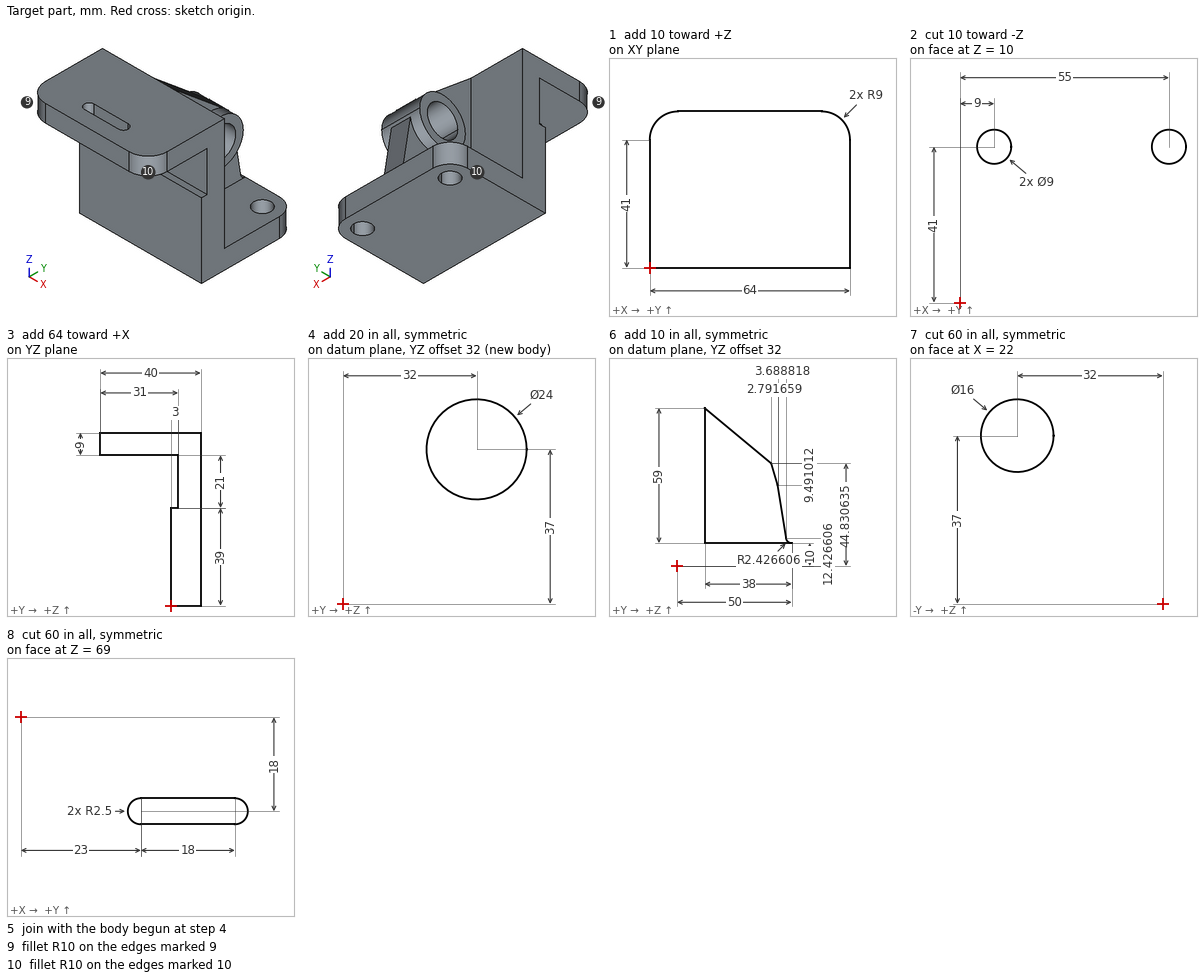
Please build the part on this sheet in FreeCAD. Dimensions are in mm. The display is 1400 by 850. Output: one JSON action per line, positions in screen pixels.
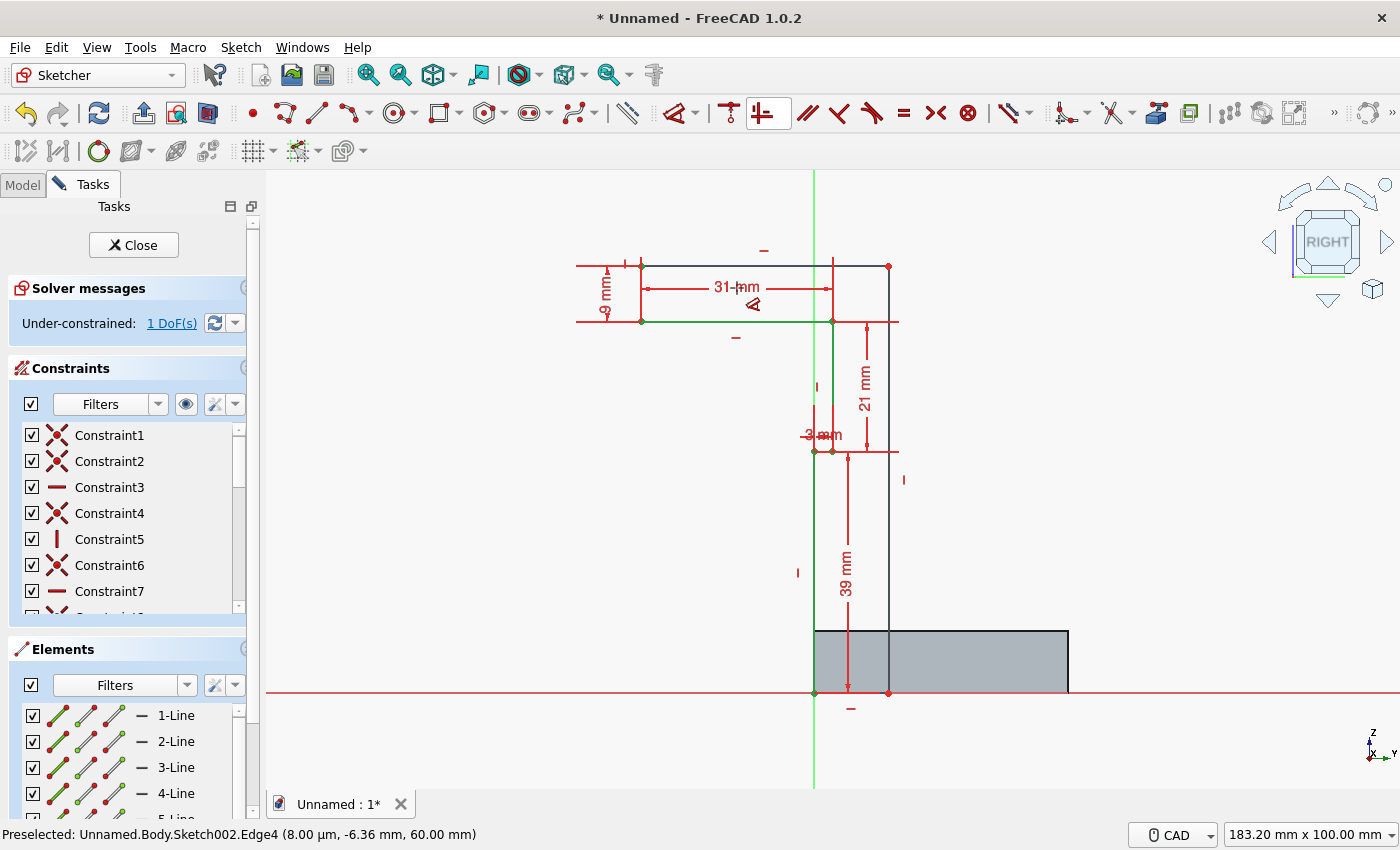
{"action": "left_click", "coordinate": [715, 266]}
{"action": "left_click", "coordinate": [765, 232]}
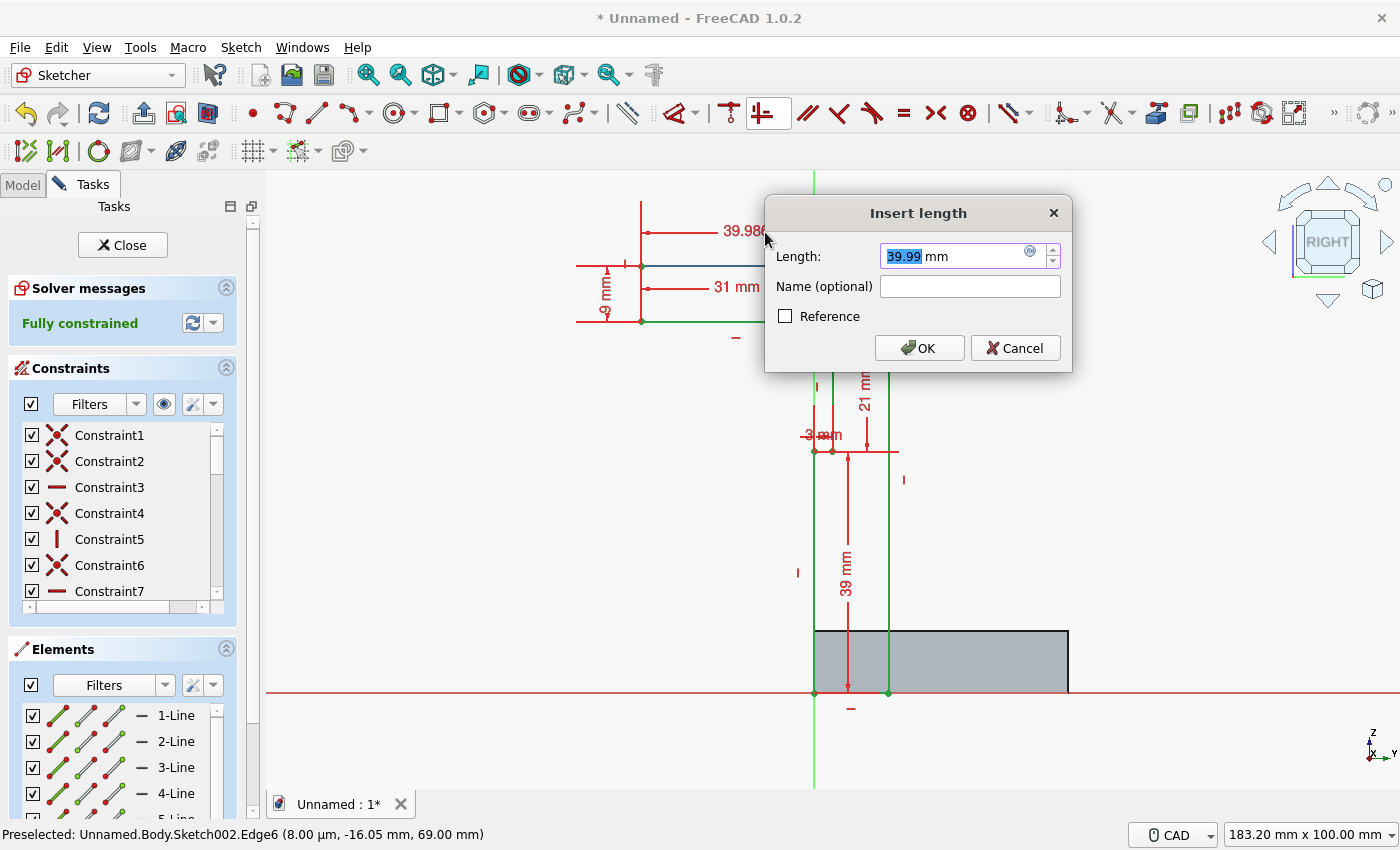
{"action": "type", "text": "40"}
{"action": "key", "text": "Return"}
{"action": "key", "text": "Escape"}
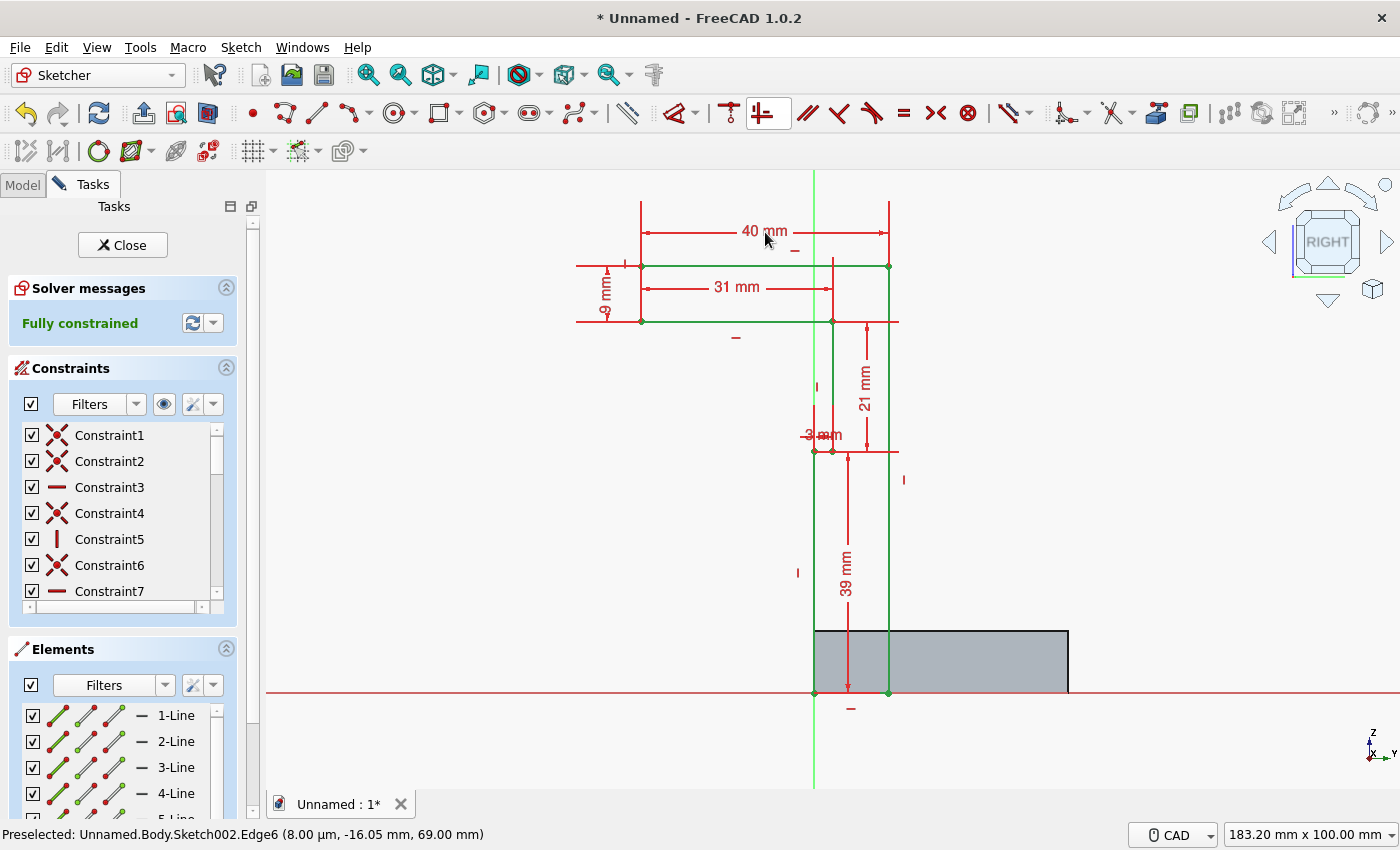
{"action": "left_click", "coordinate": [123, 245]}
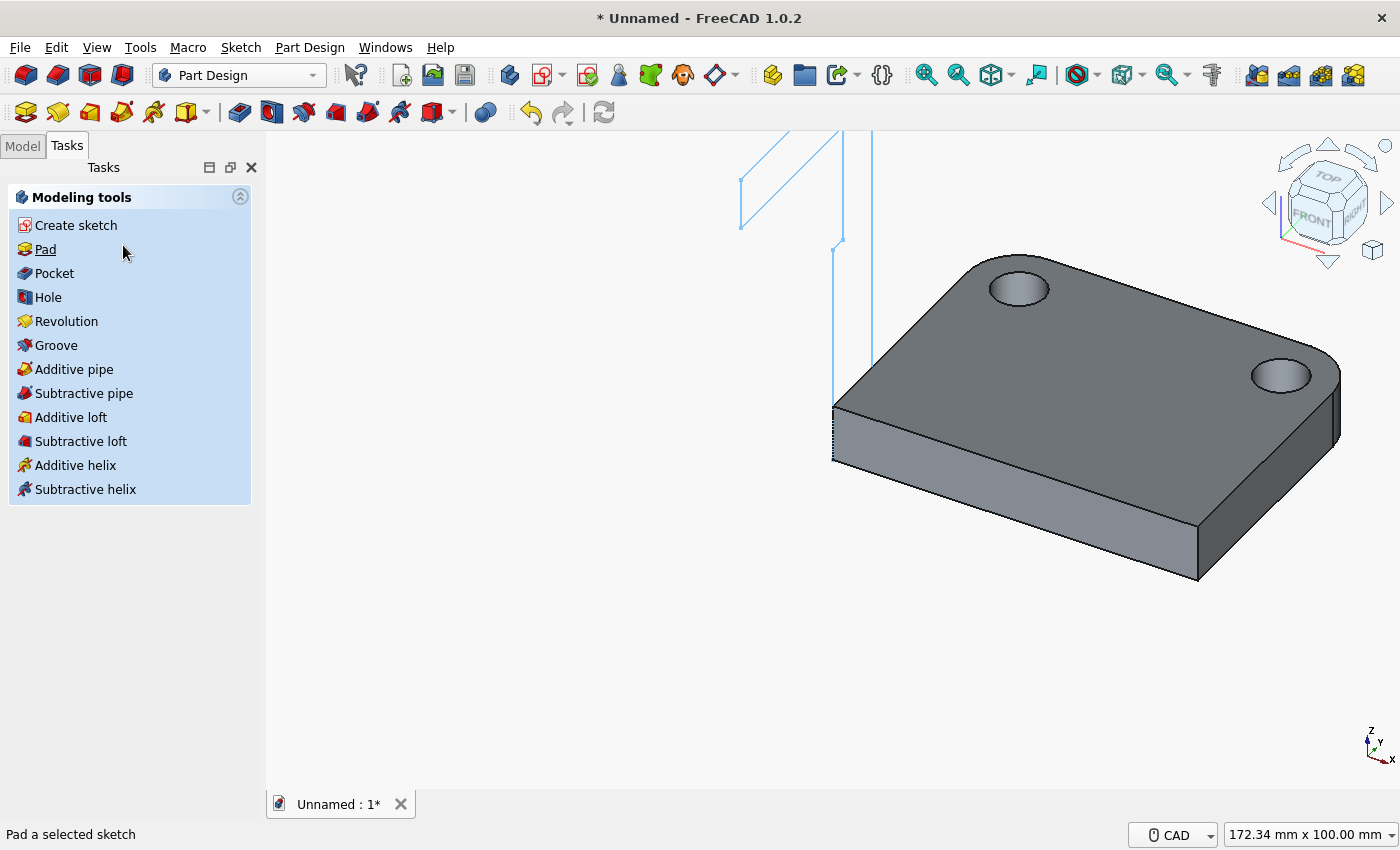
{"action": "left_click", "coordinate": [26, 112]}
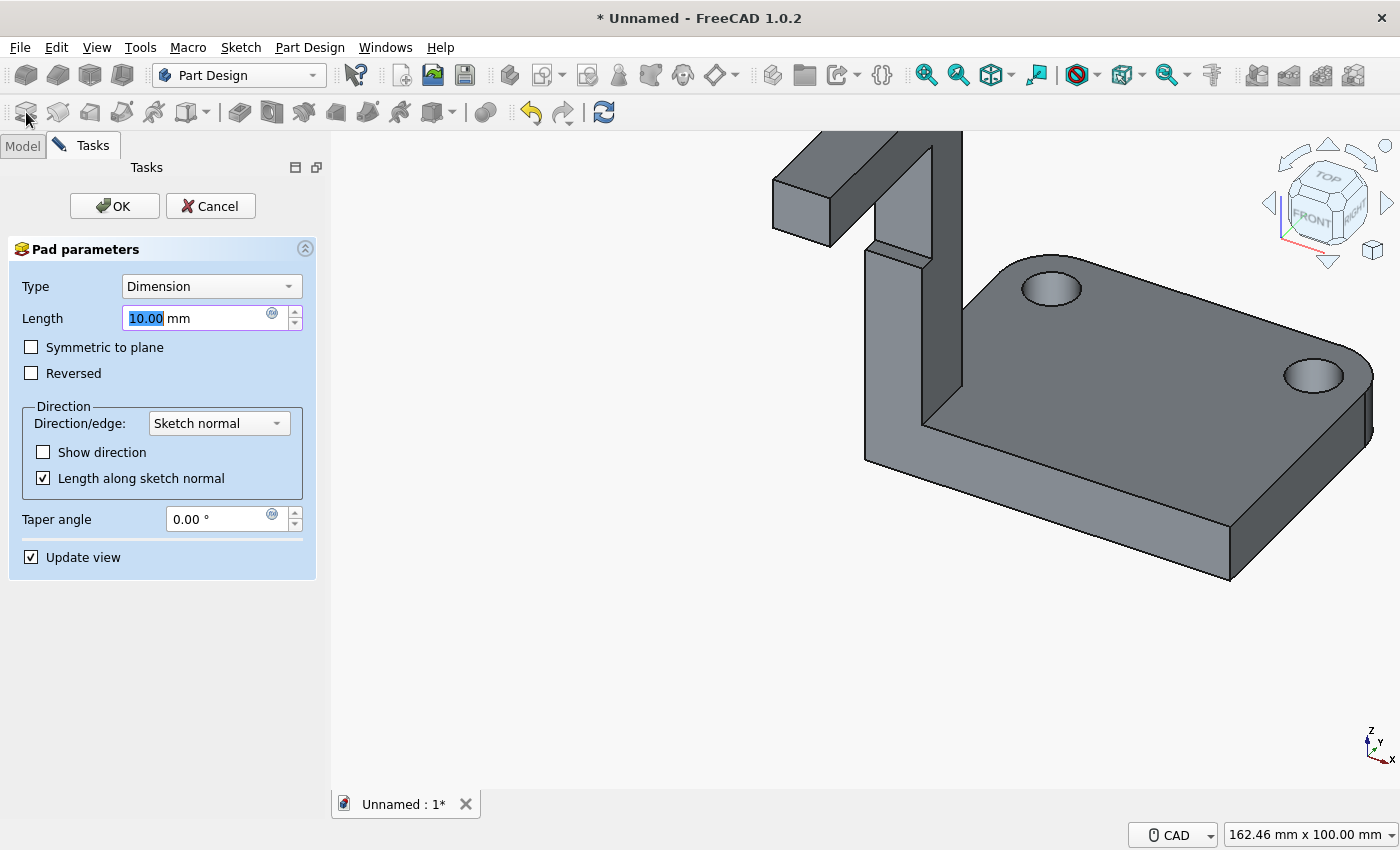
{"action": "type", "text": "64"}
{"action": "key", "text": "Tab"}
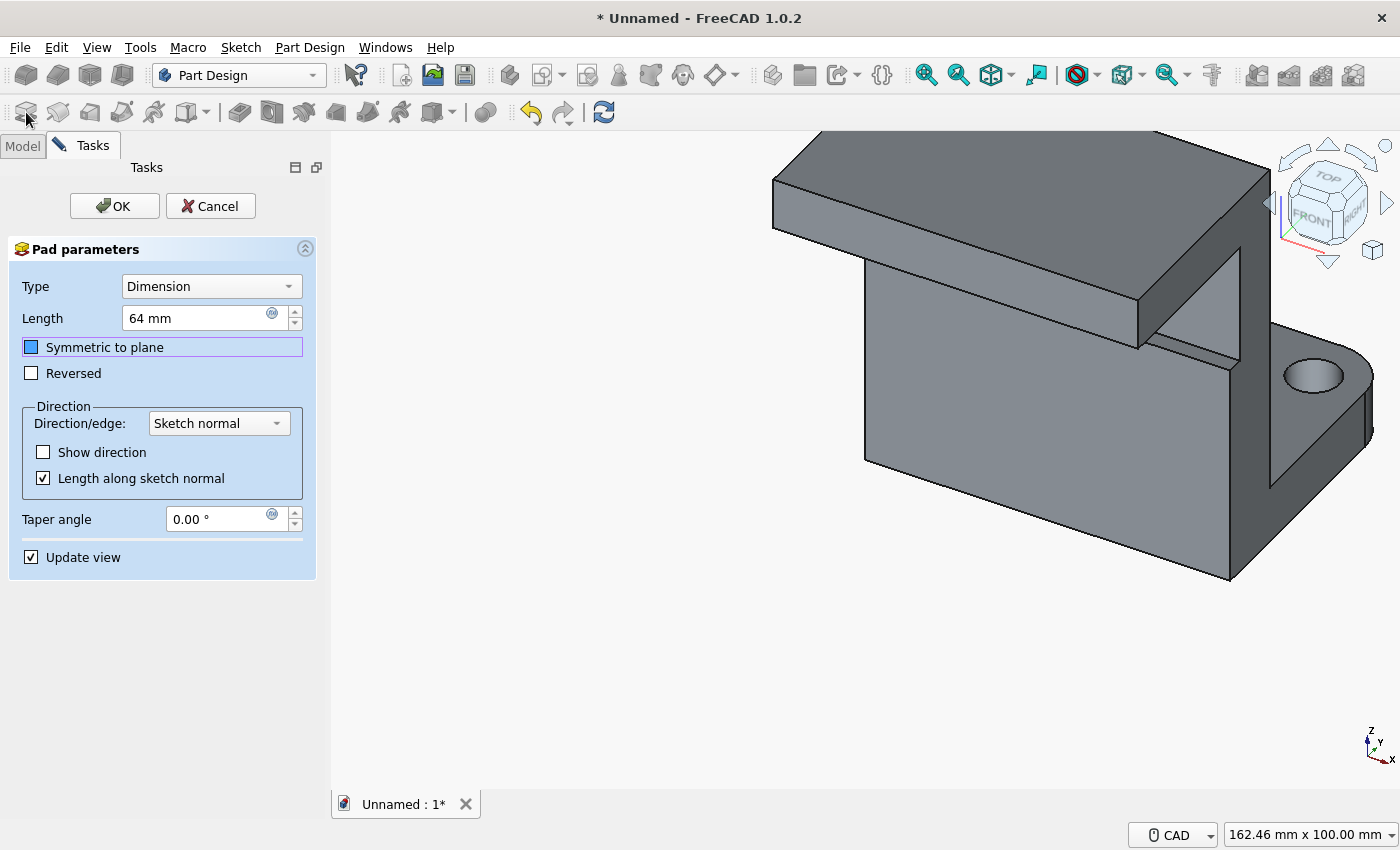
{"action": "left_click", "coordinate": [115, 206]}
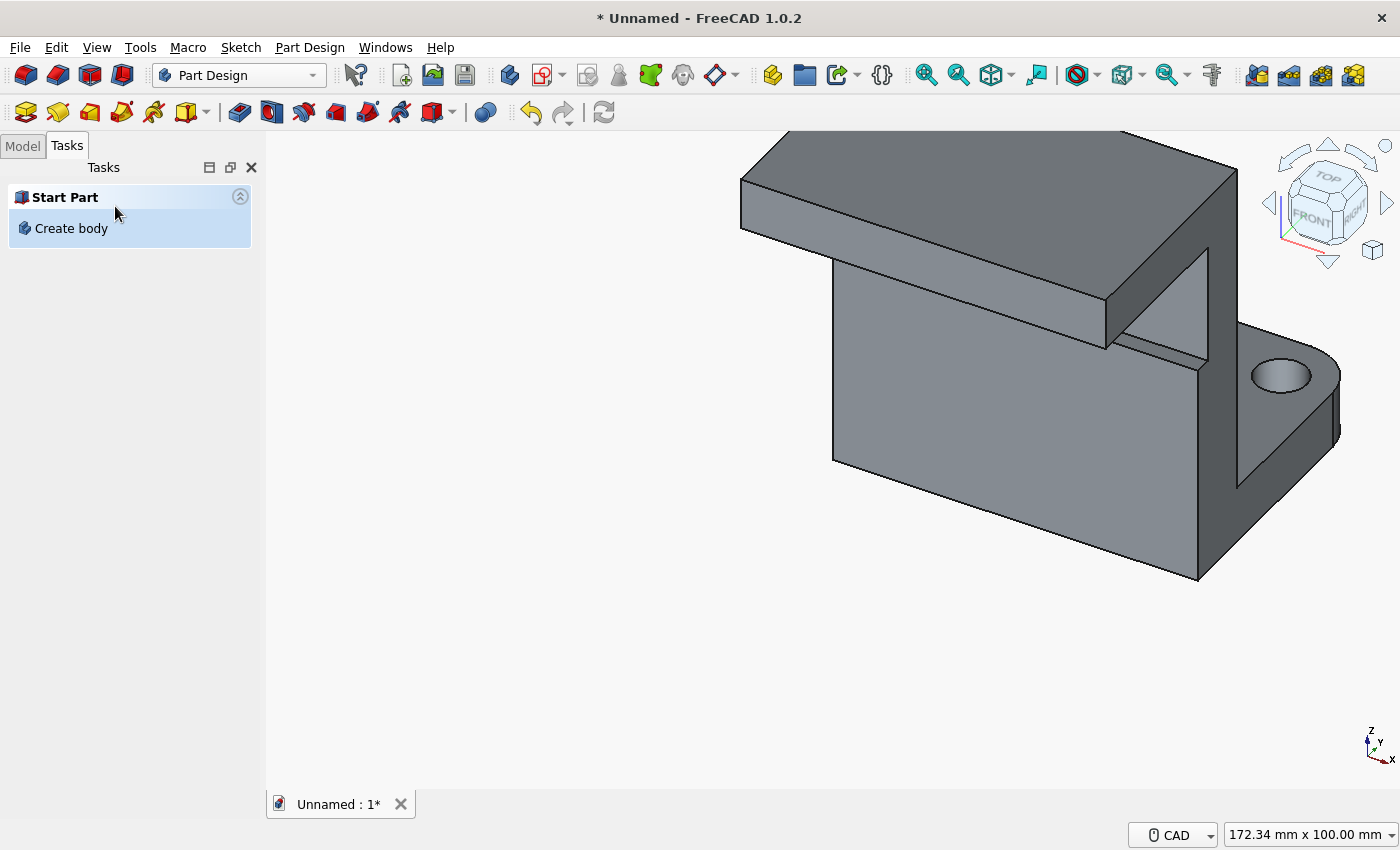
{"action": "left_click", "coordinate": [928, 76]}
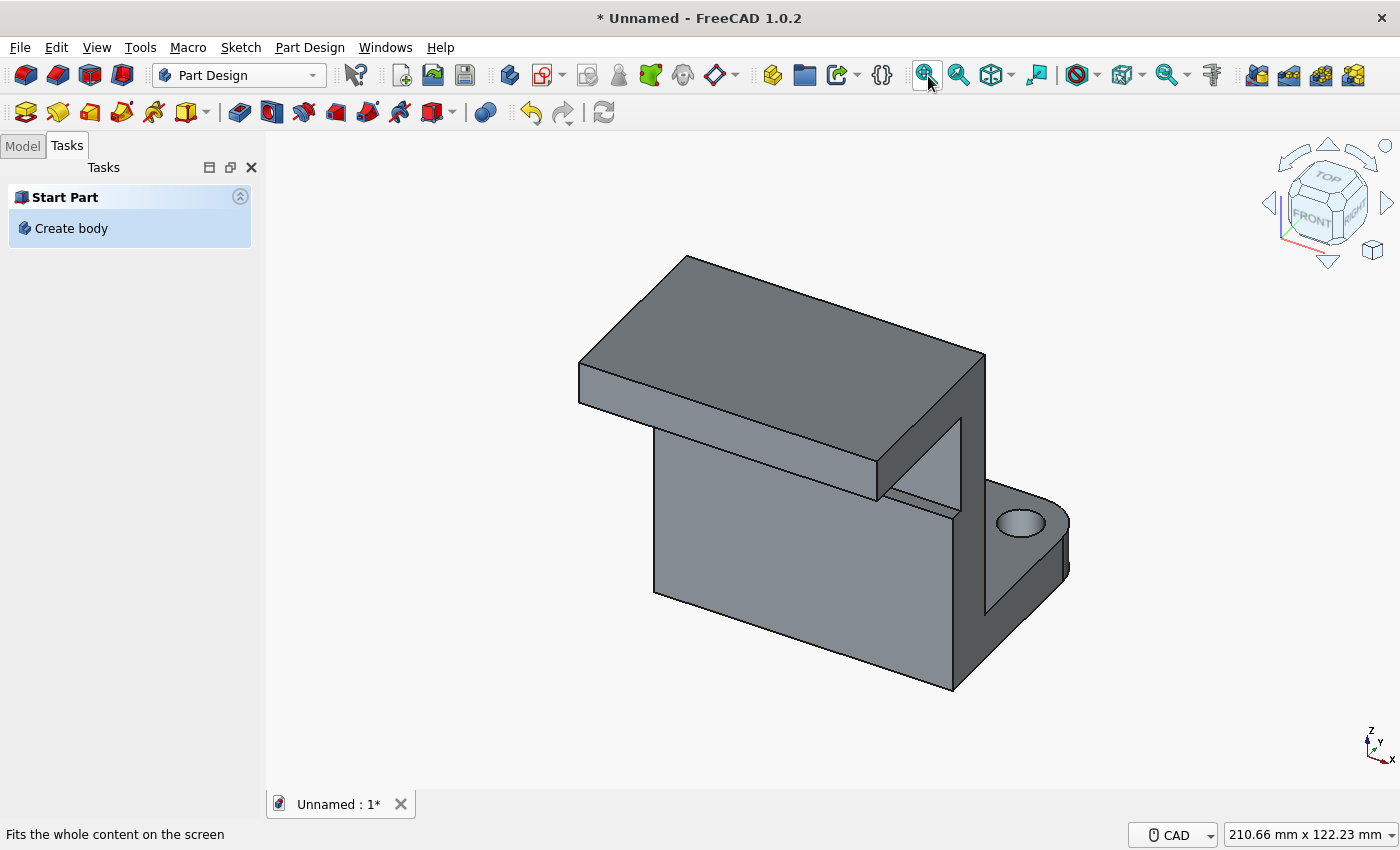
{"action": "left_click", "coordinate": [510, 76]}